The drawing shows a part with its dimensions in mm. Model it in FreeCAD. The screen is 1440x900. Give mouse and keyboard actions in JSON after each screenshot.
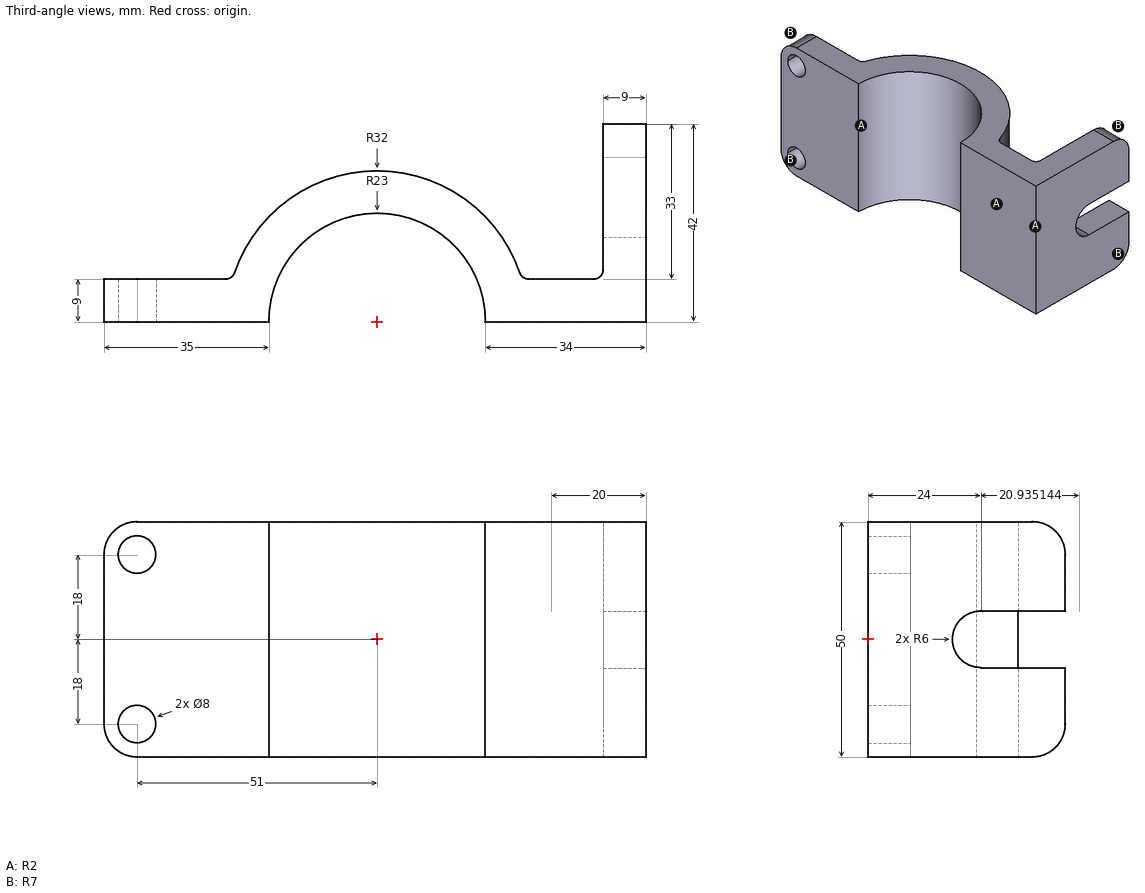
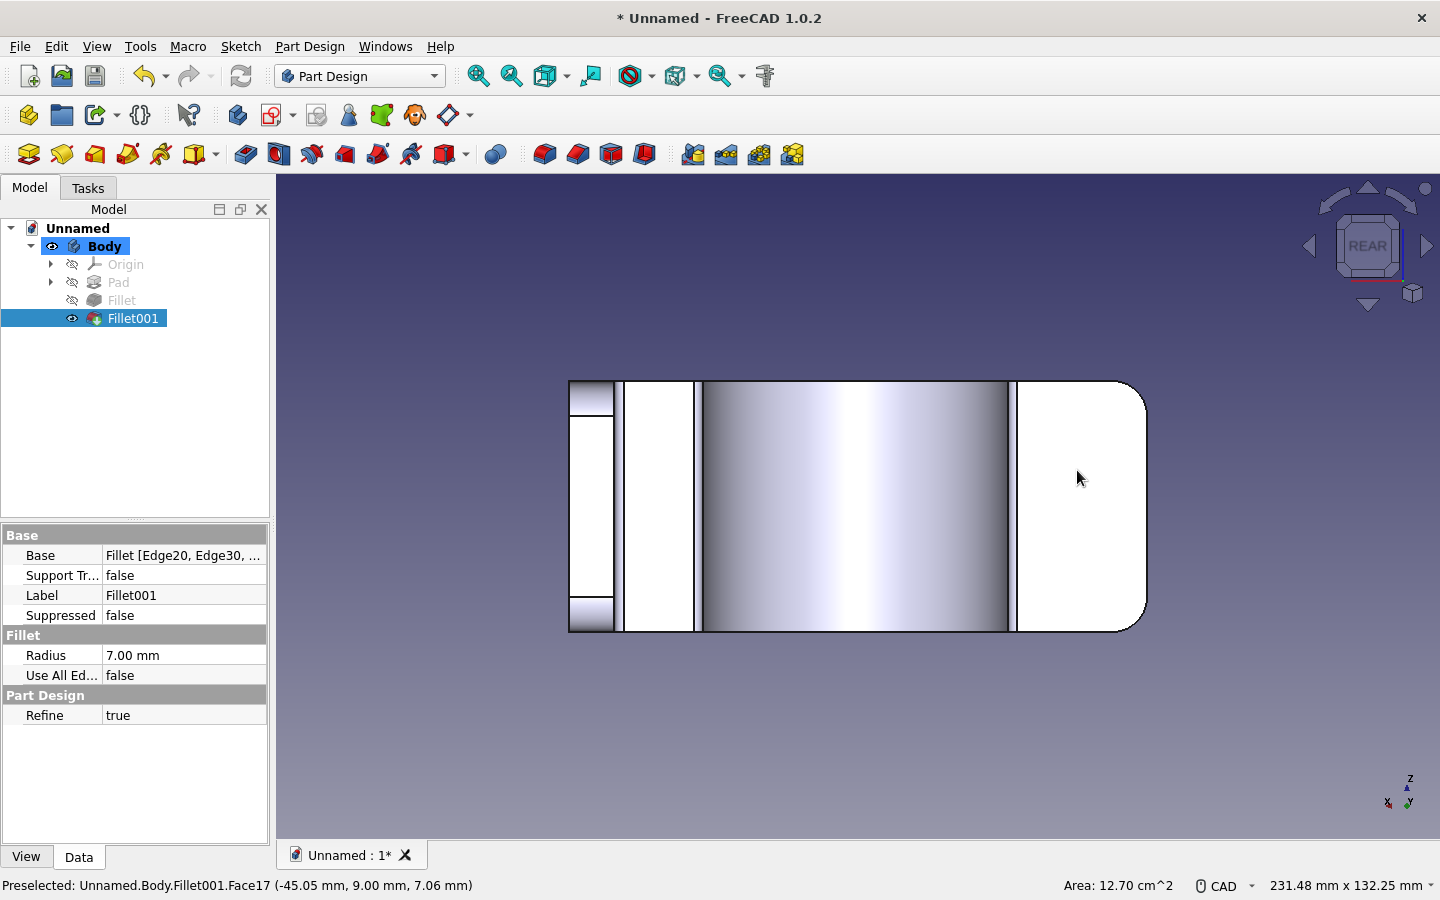
{"action": "left_click", "coordinate": [270, 116]}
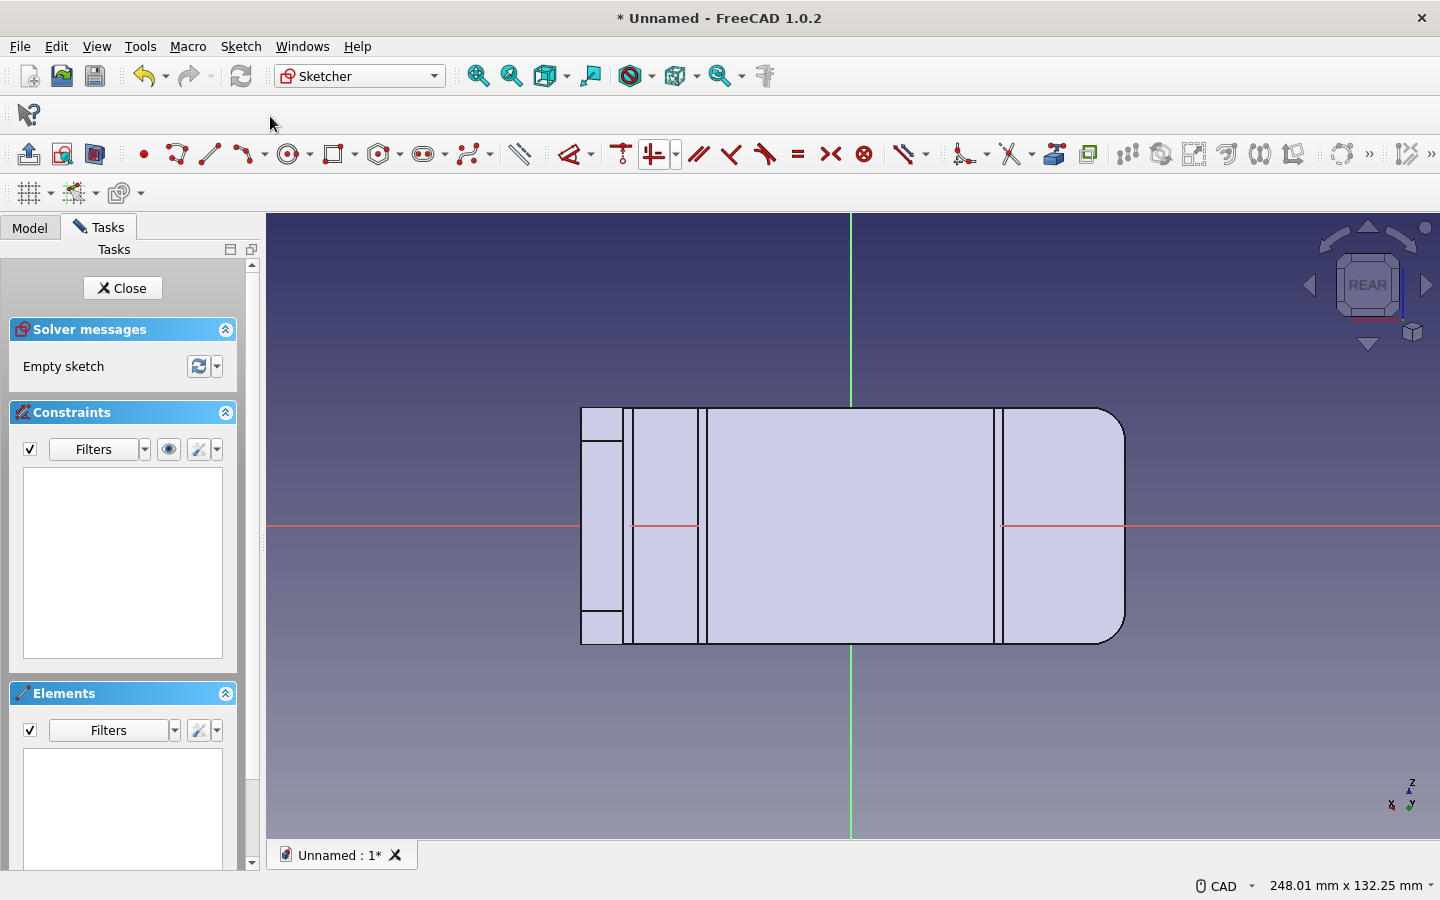
{"action": "left_click", "coordinate": [95, 154]}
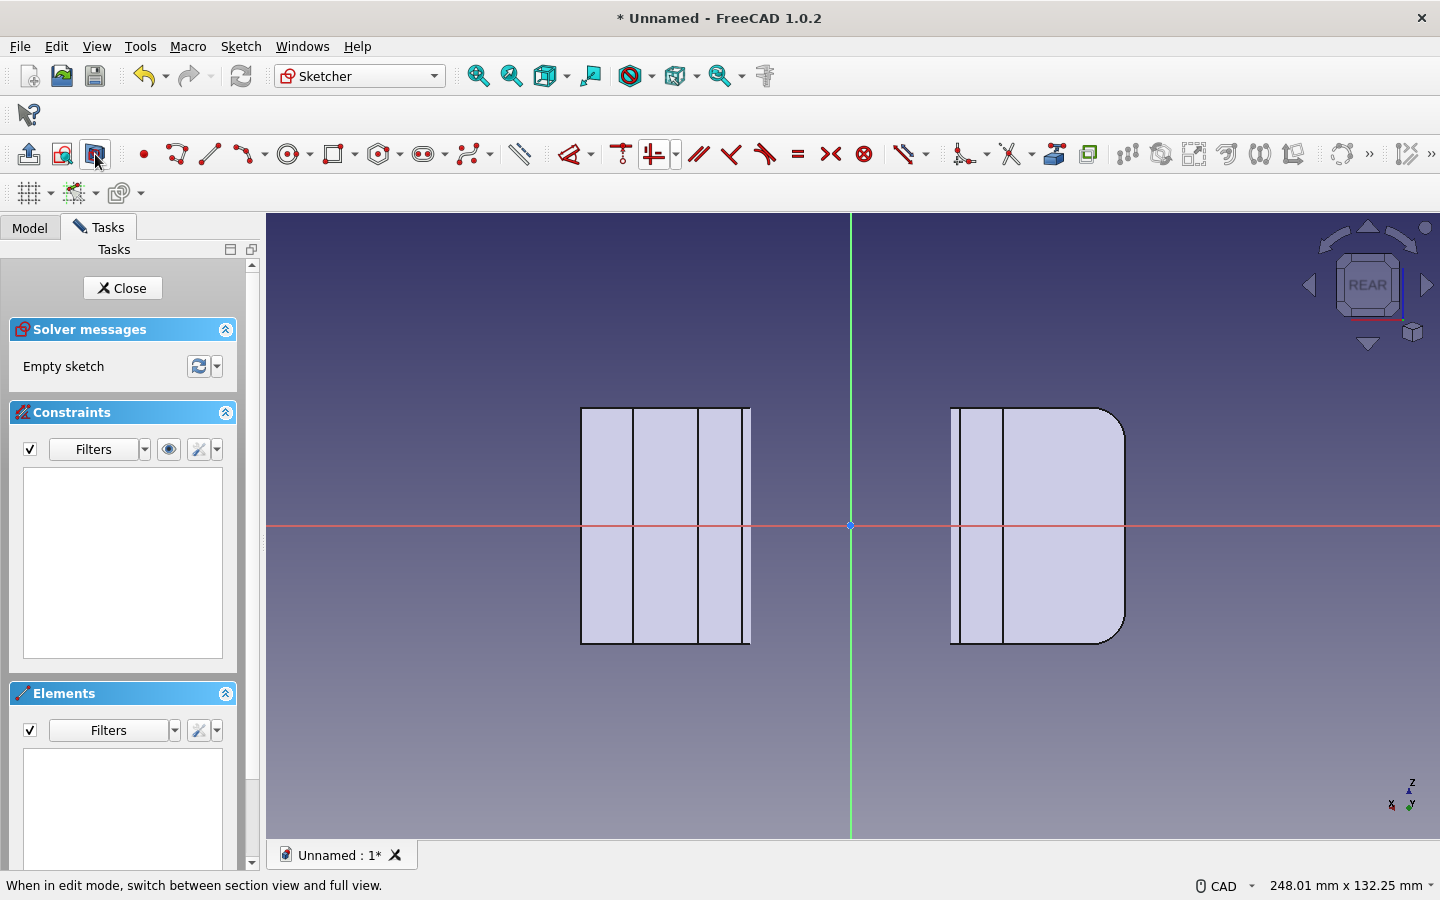
{"action": "scroll", "coordinate": [1220, 526], "scroll_direction": "up", "scroll_amount": 3}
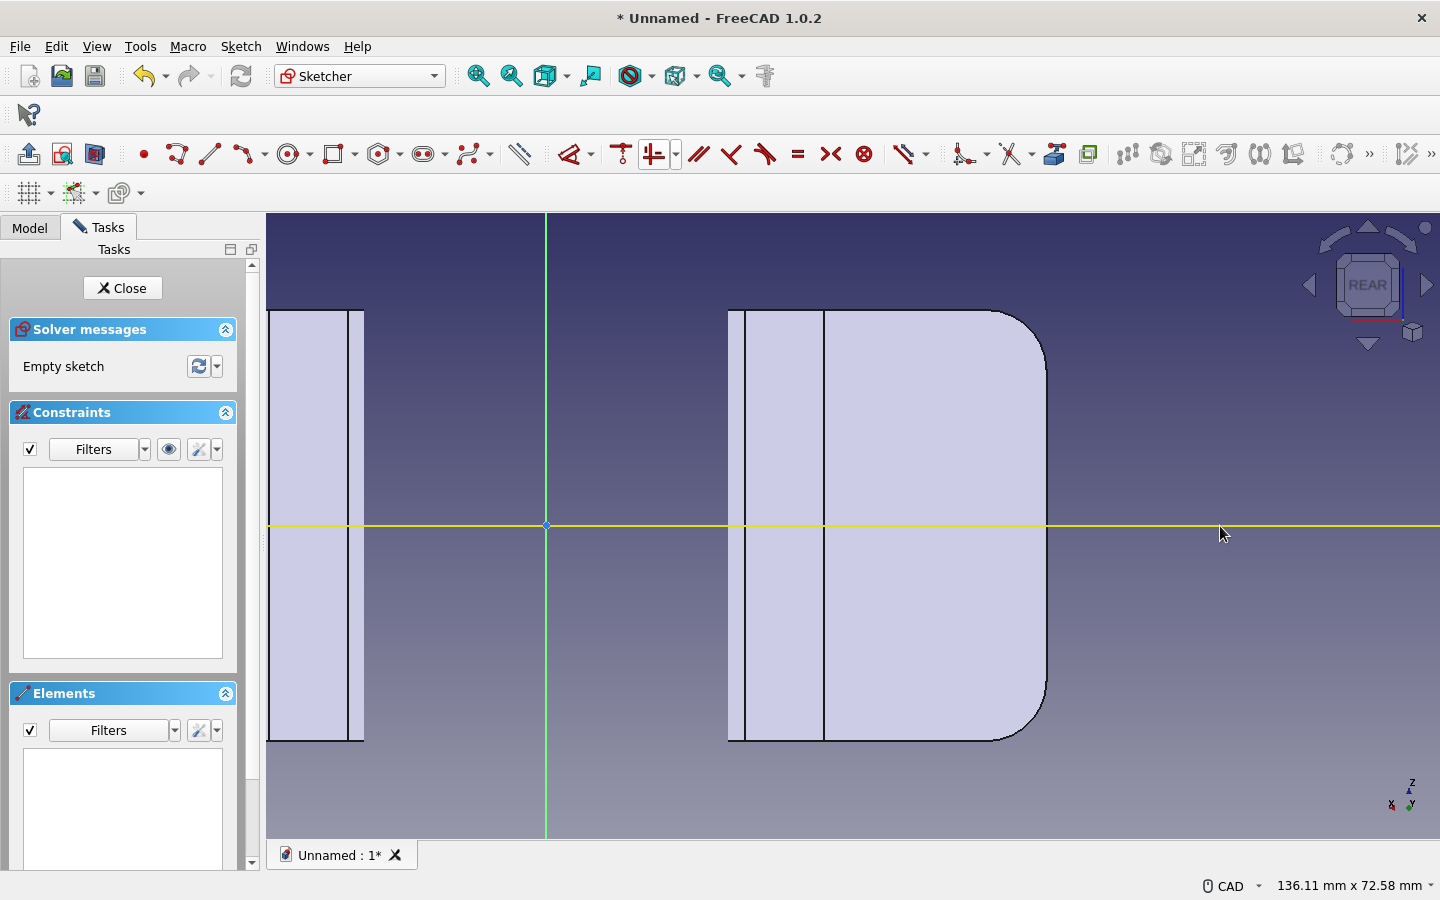
{"action": "left_click", "coordinate": [288, 154]}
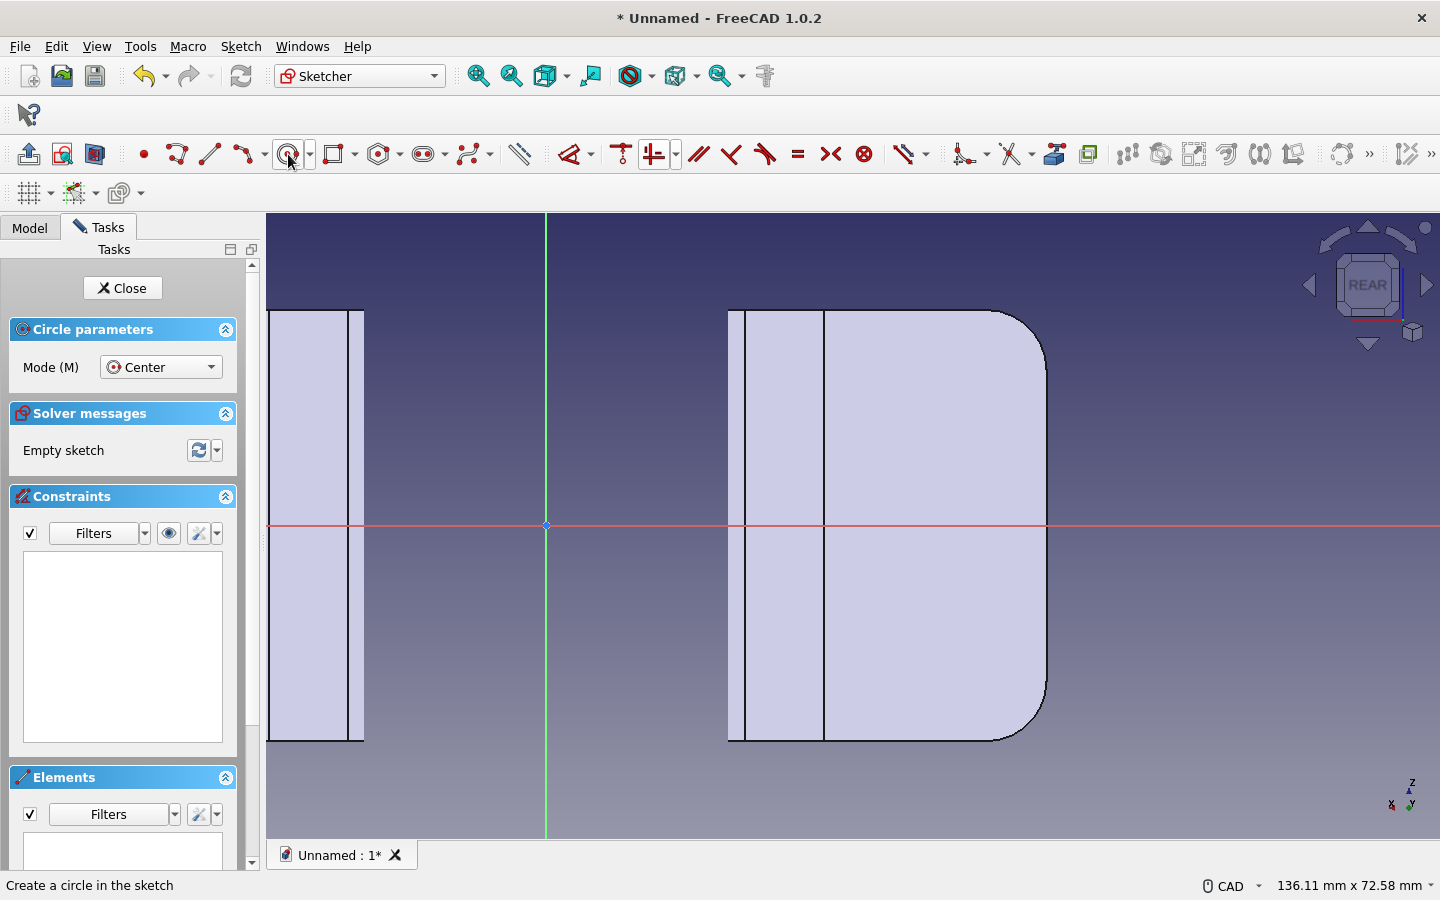
{"action": "left_click", "coordinate": [986, 681]}
{"action": "mouse_move", "coordinate": [1011, 656]}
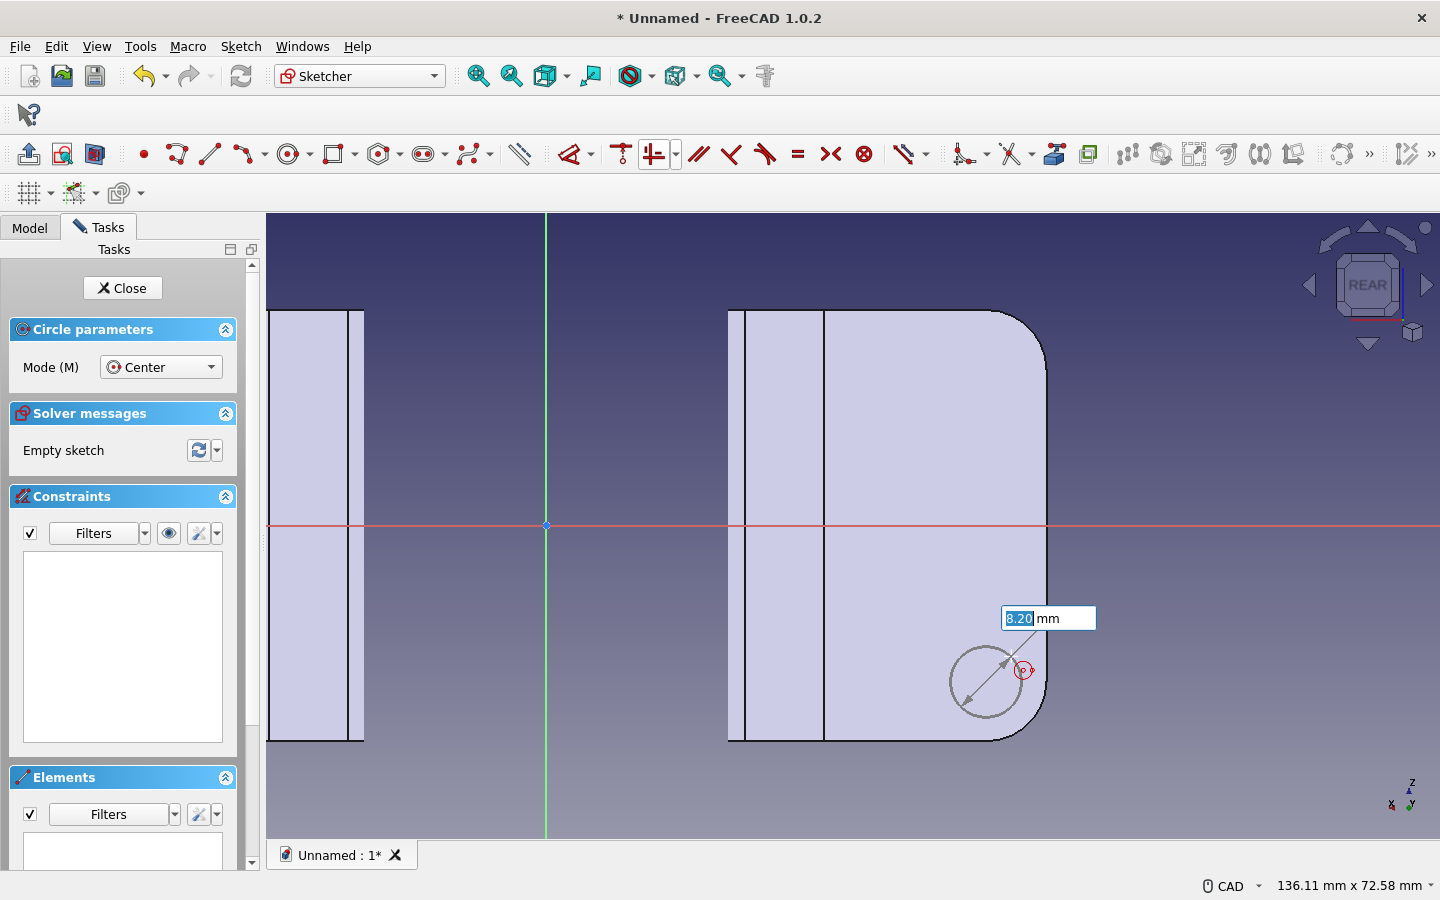
{"action": "type", "text": "8"}
{"action": "key", "text": "Return"}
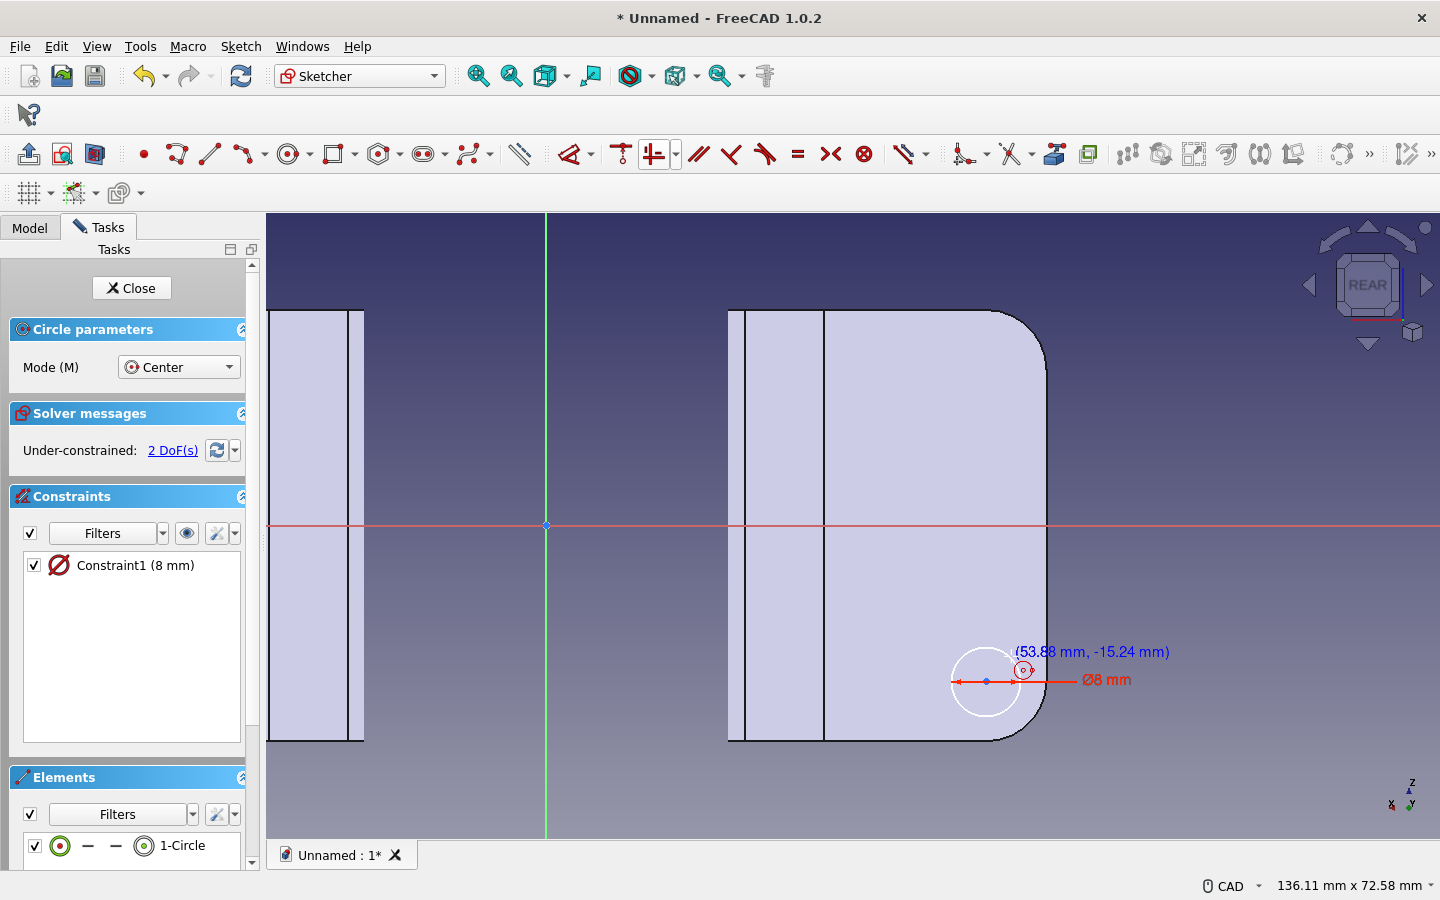
{"action": "left_click", "coordinate": [986, 370]}
{"action": "mouse_move", "coordinate": [1011, 346]}